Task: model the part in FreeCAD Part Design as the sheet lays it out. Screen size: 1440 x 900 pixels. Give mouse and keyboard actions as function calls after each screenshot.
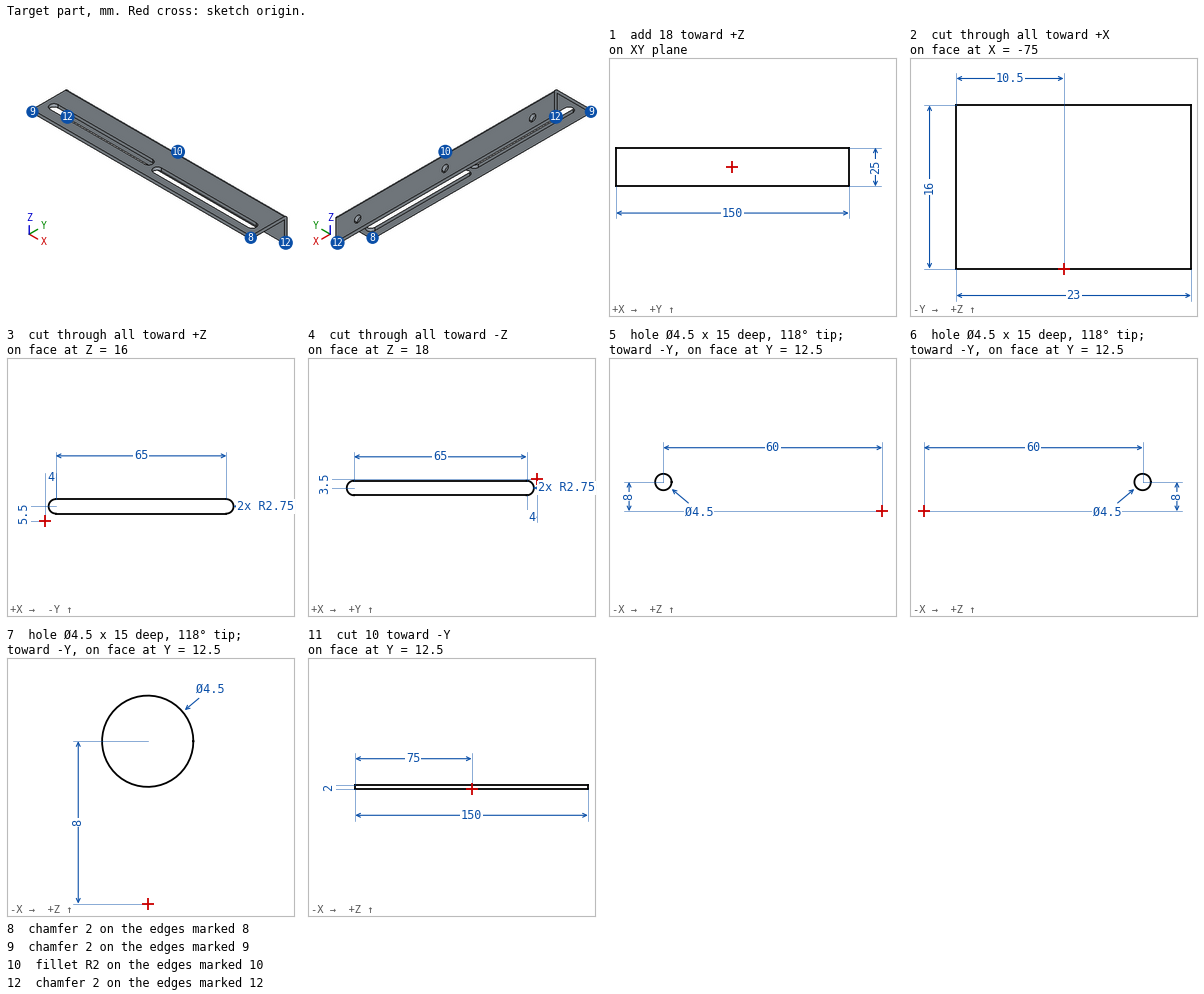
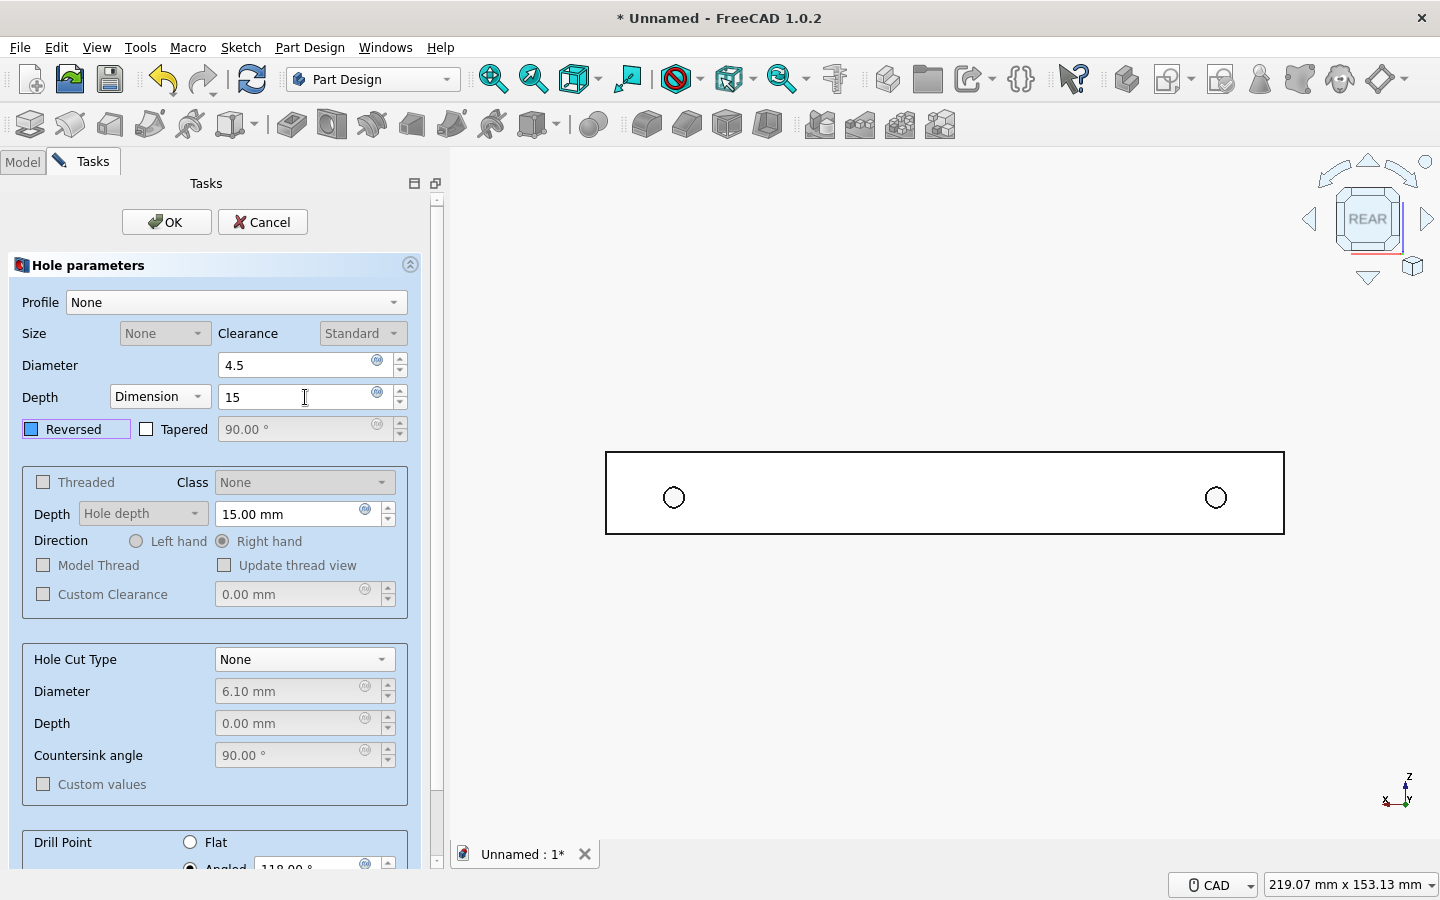
click(167, 222)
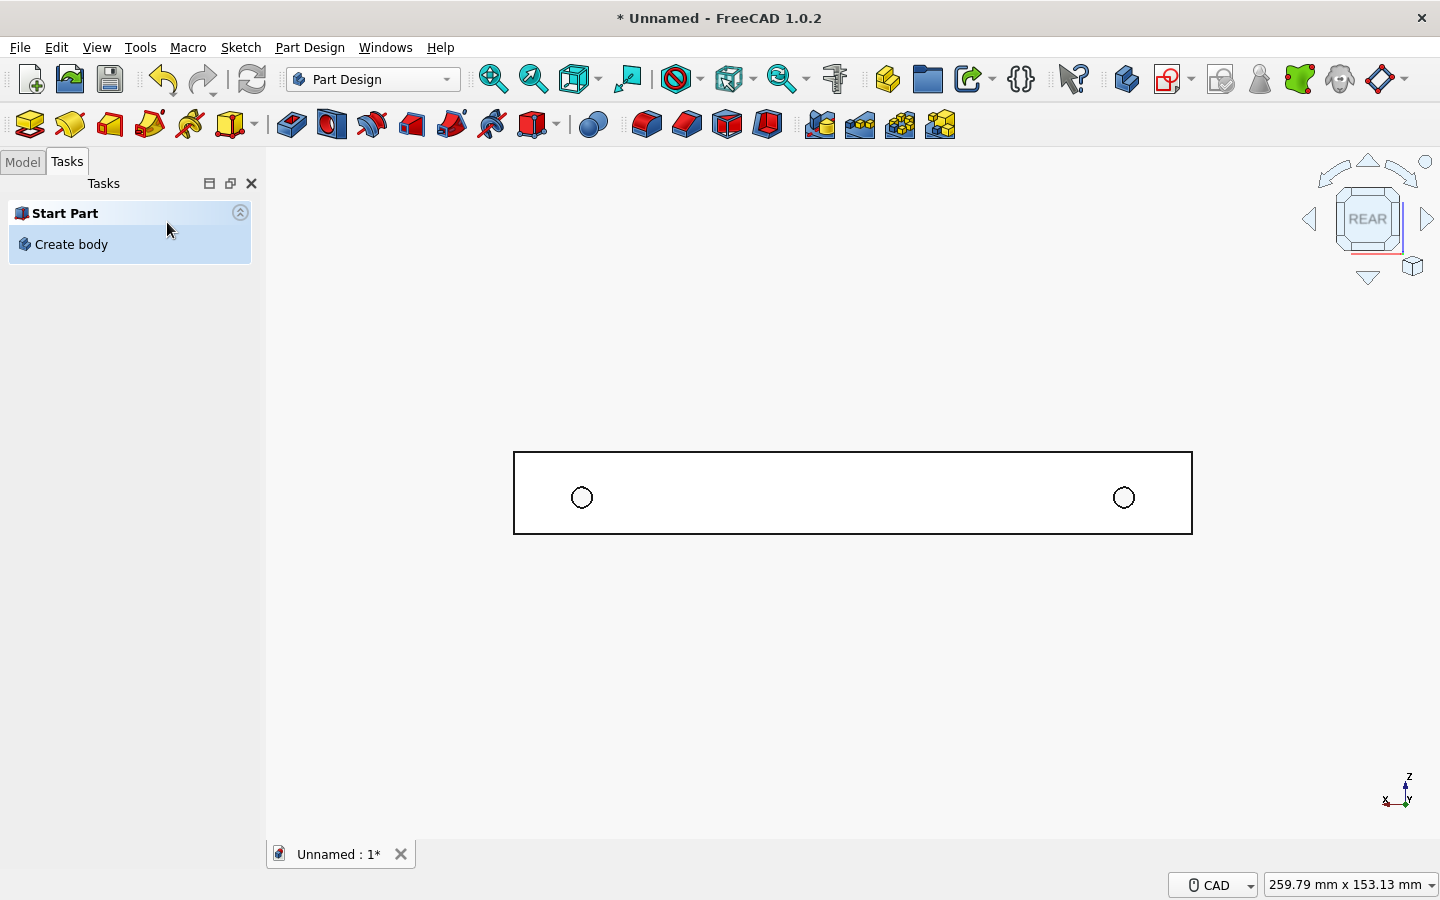
click(659, 492)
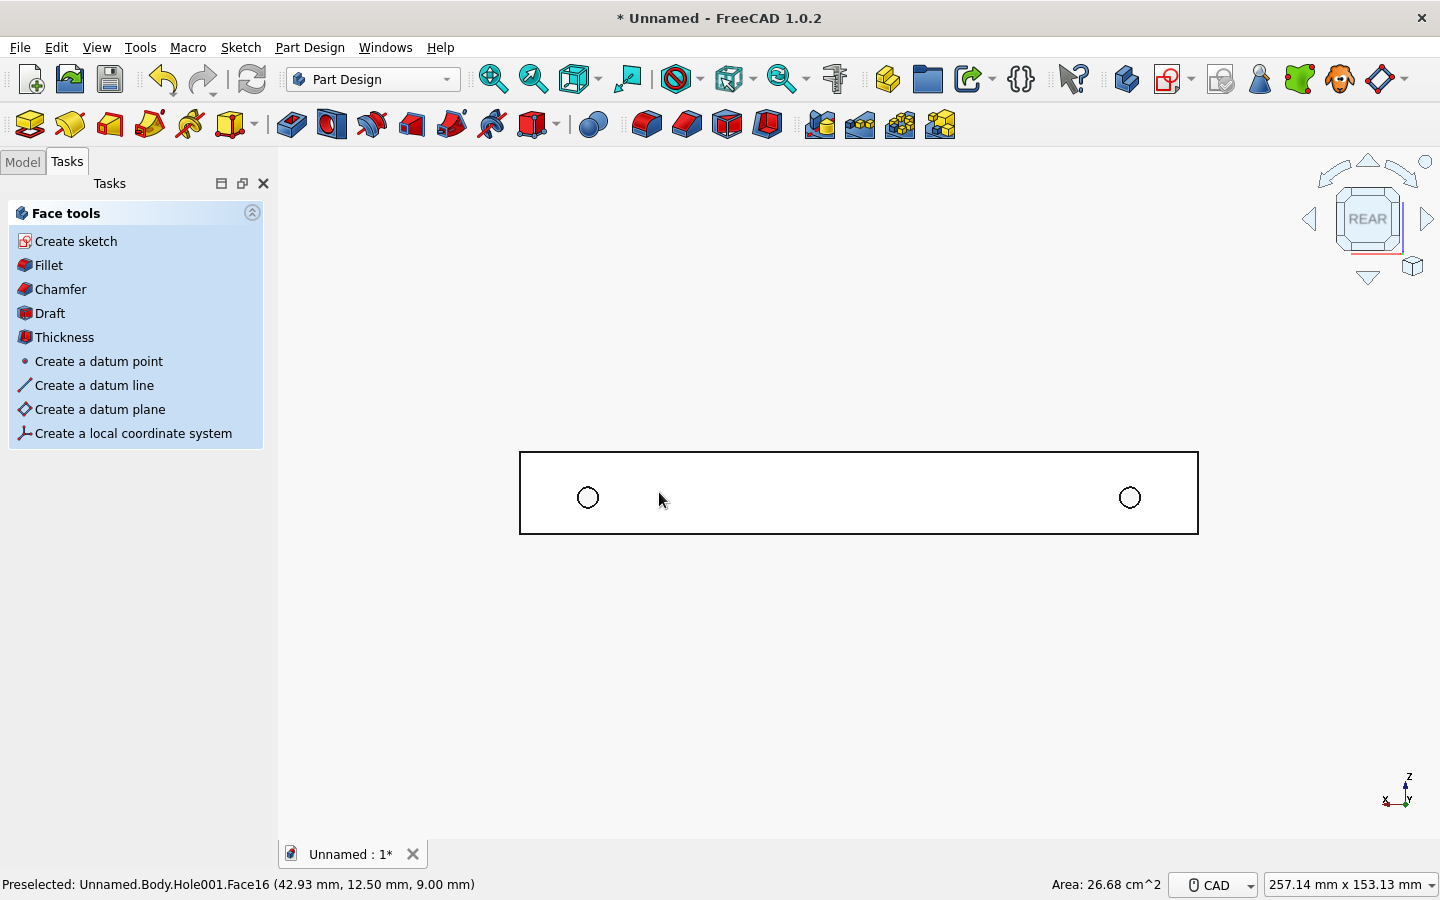
click(1168, 80)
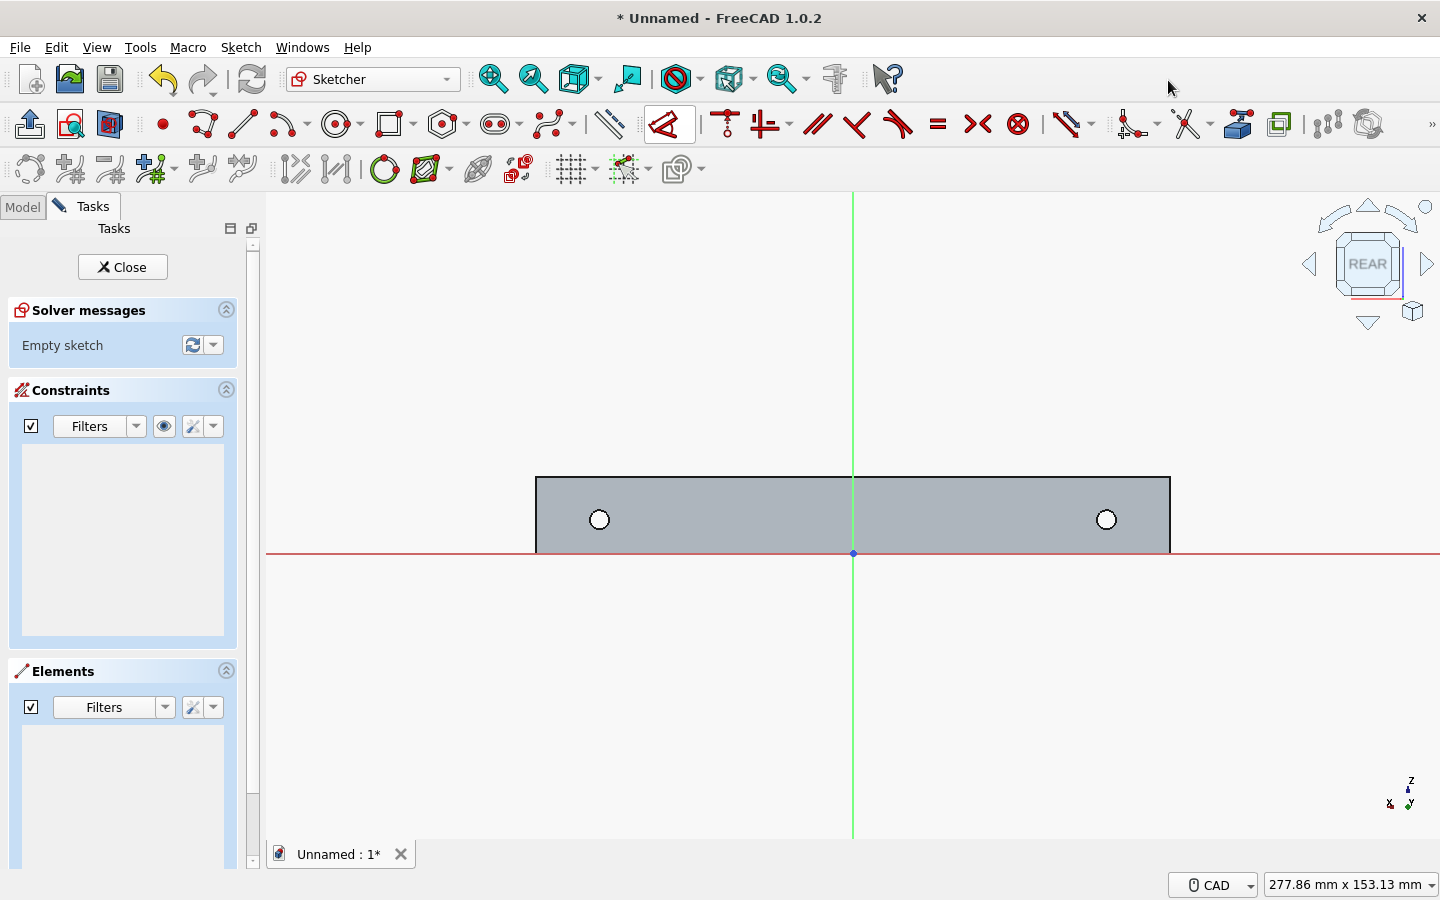
scroll(862, 534, up, 11)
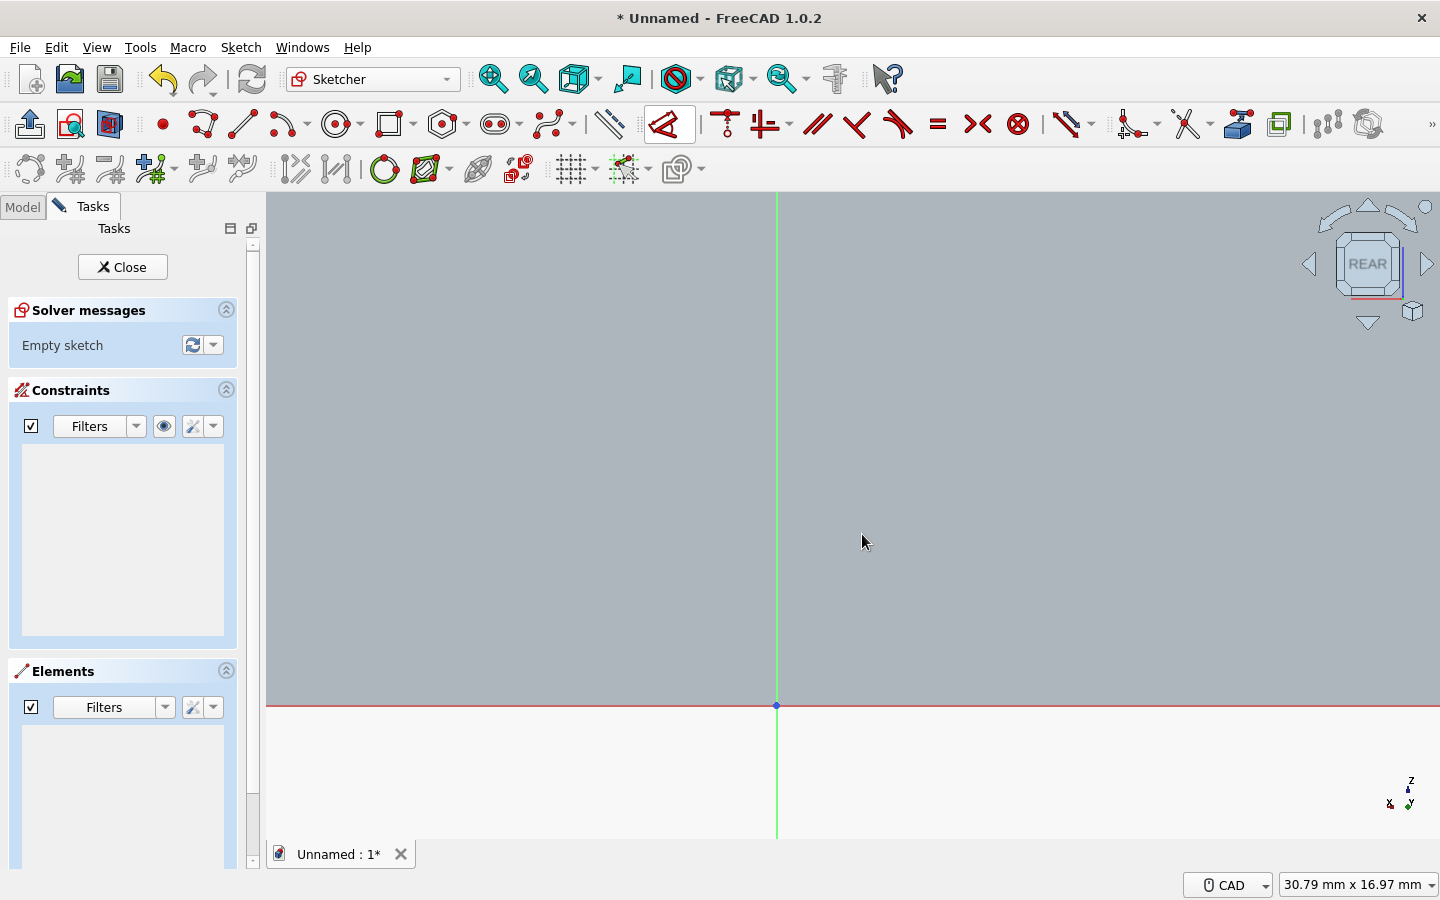
click(336, 124)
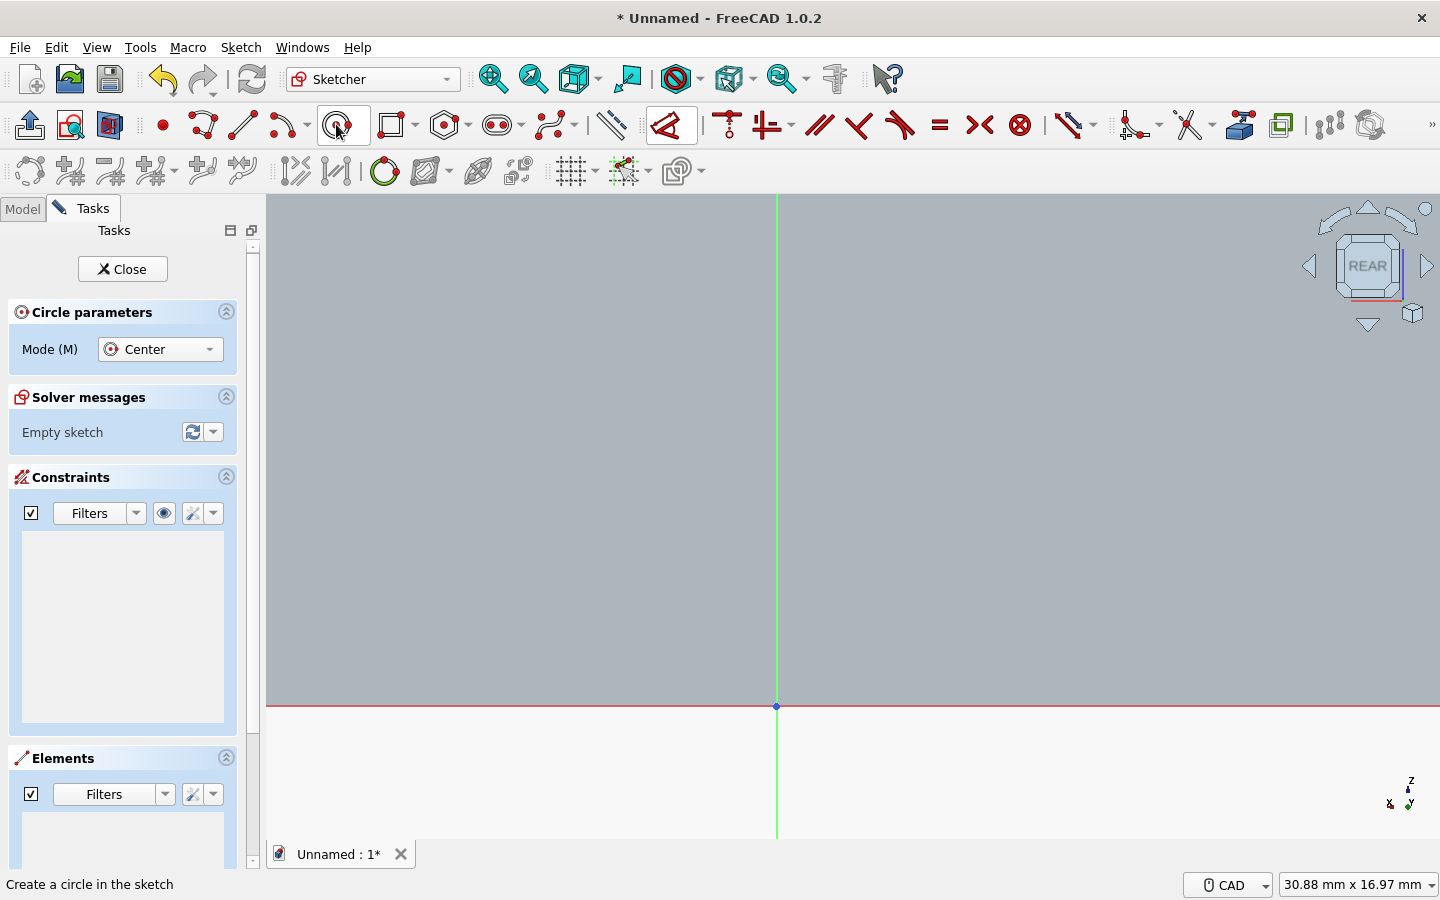
click(777, 402)
move(837, 342)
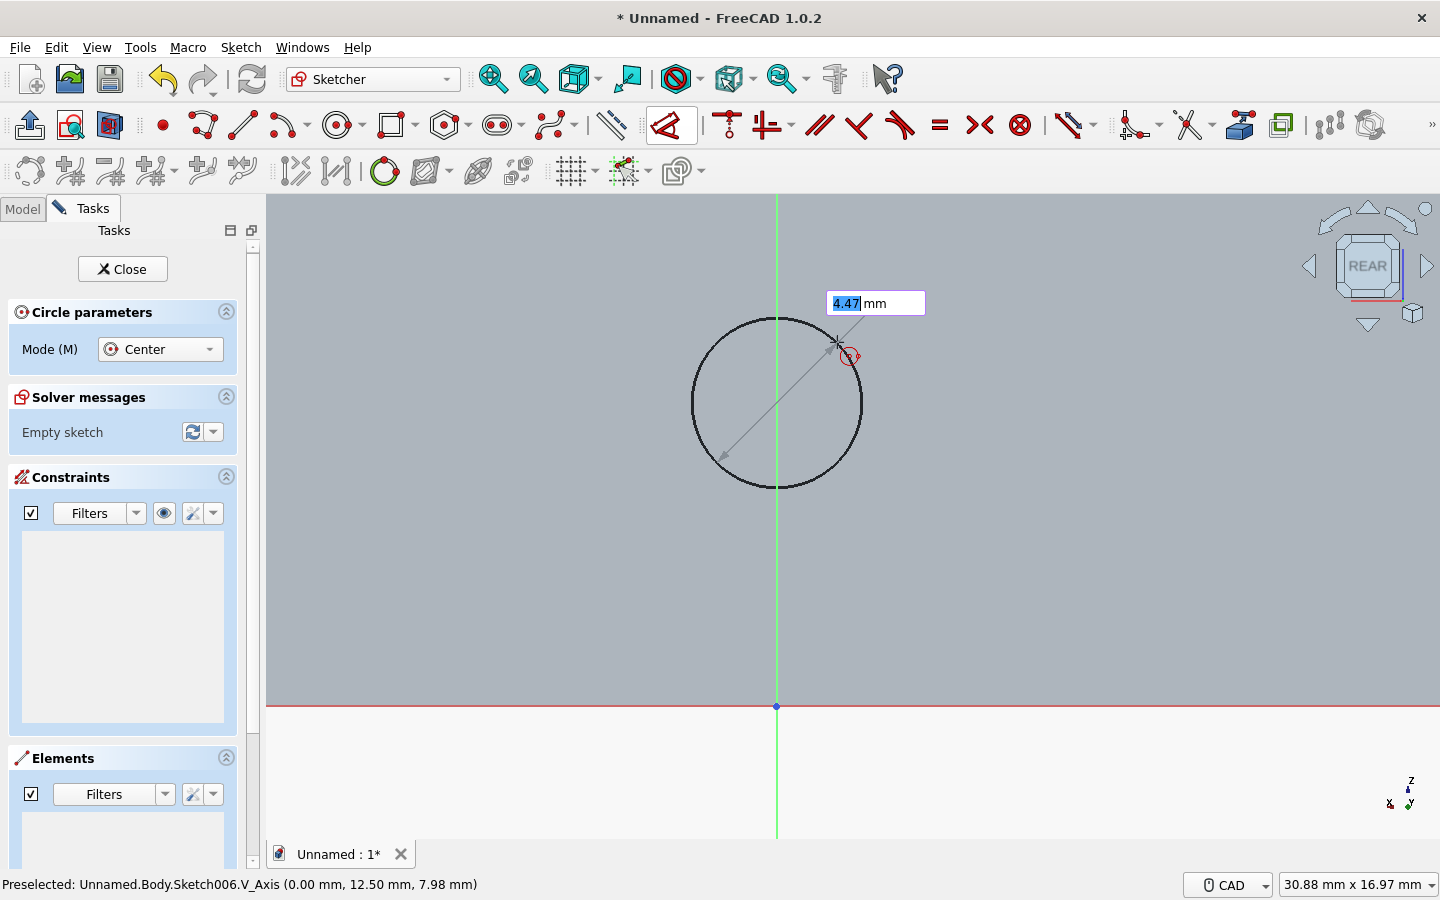
text(4.5)
key(Return)
key(Escape)